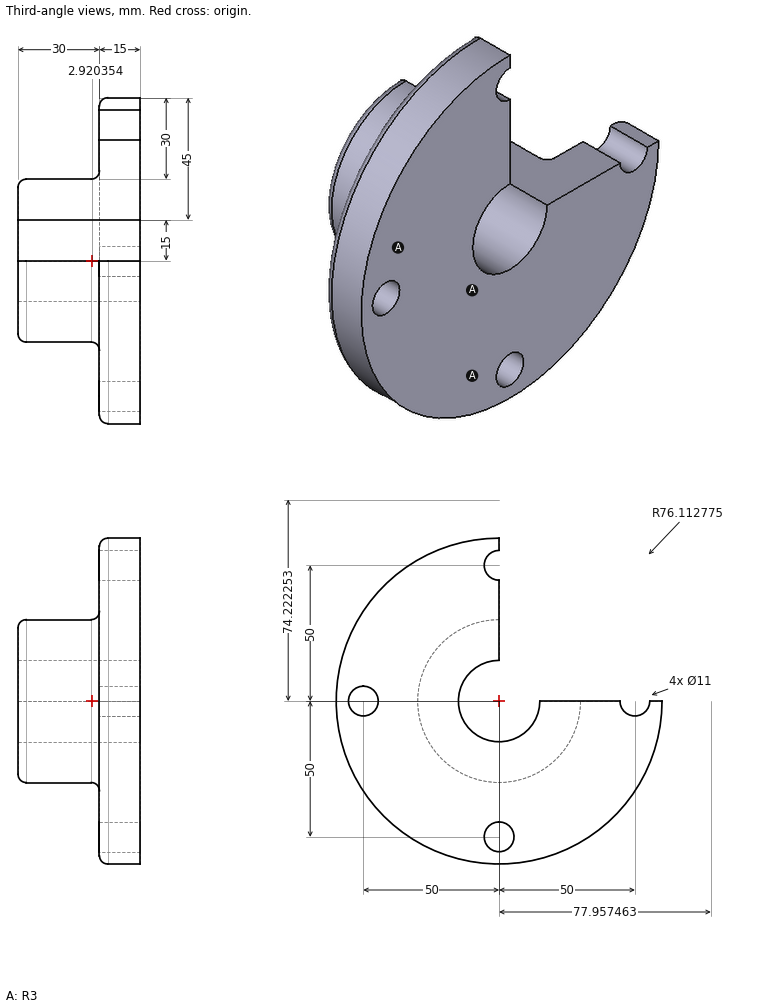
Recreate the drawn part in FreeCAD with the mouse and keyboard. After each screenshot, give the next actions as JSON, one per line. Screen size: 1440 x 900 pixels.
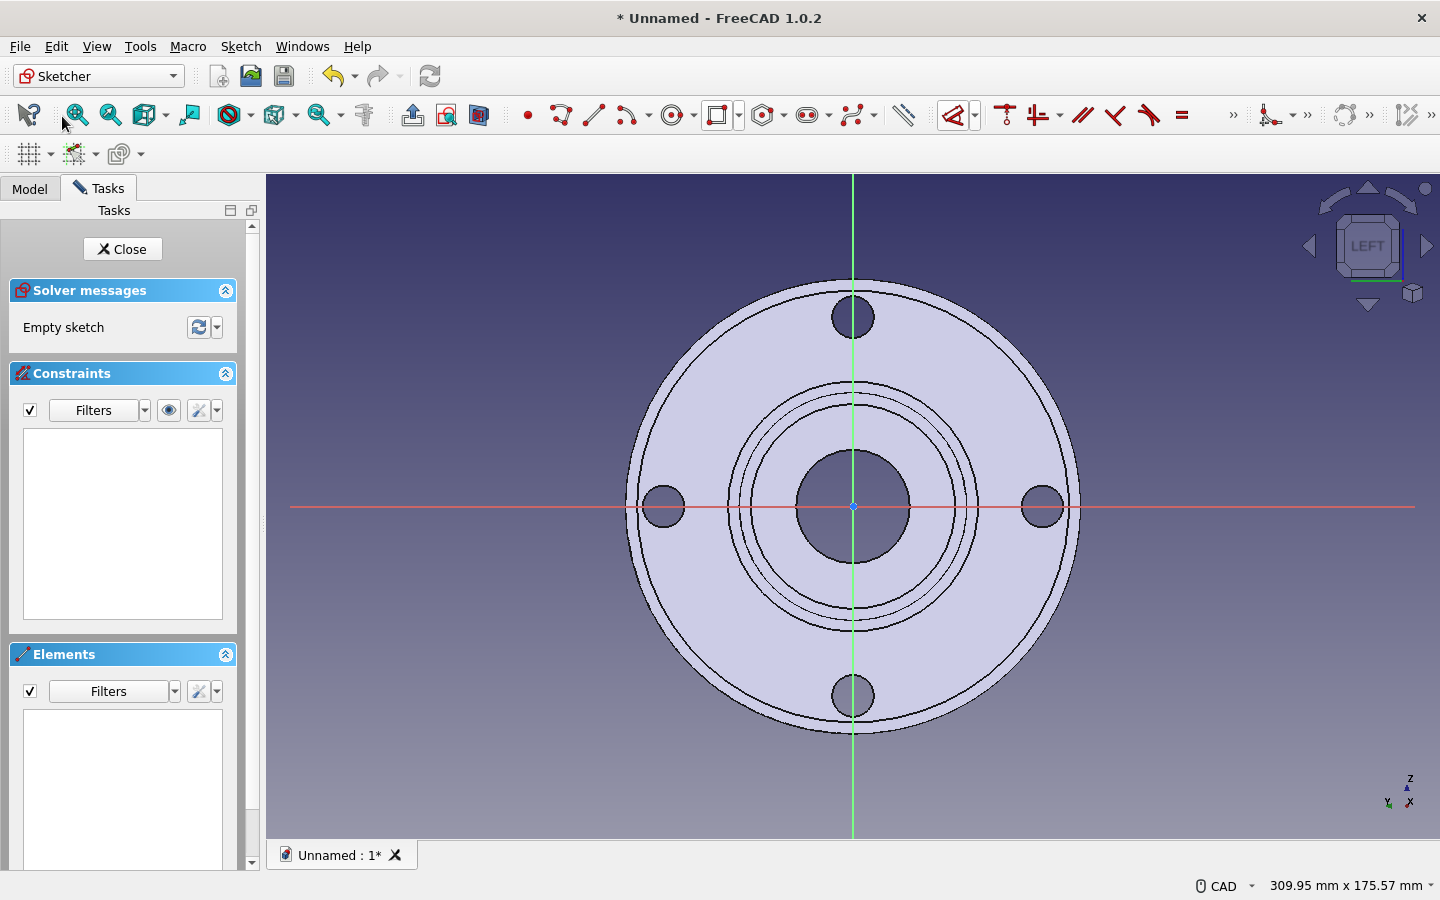
{"action": "scroll", "coordinate": [544, 202], "scroll_direction": "up", "scroll_amount": 2}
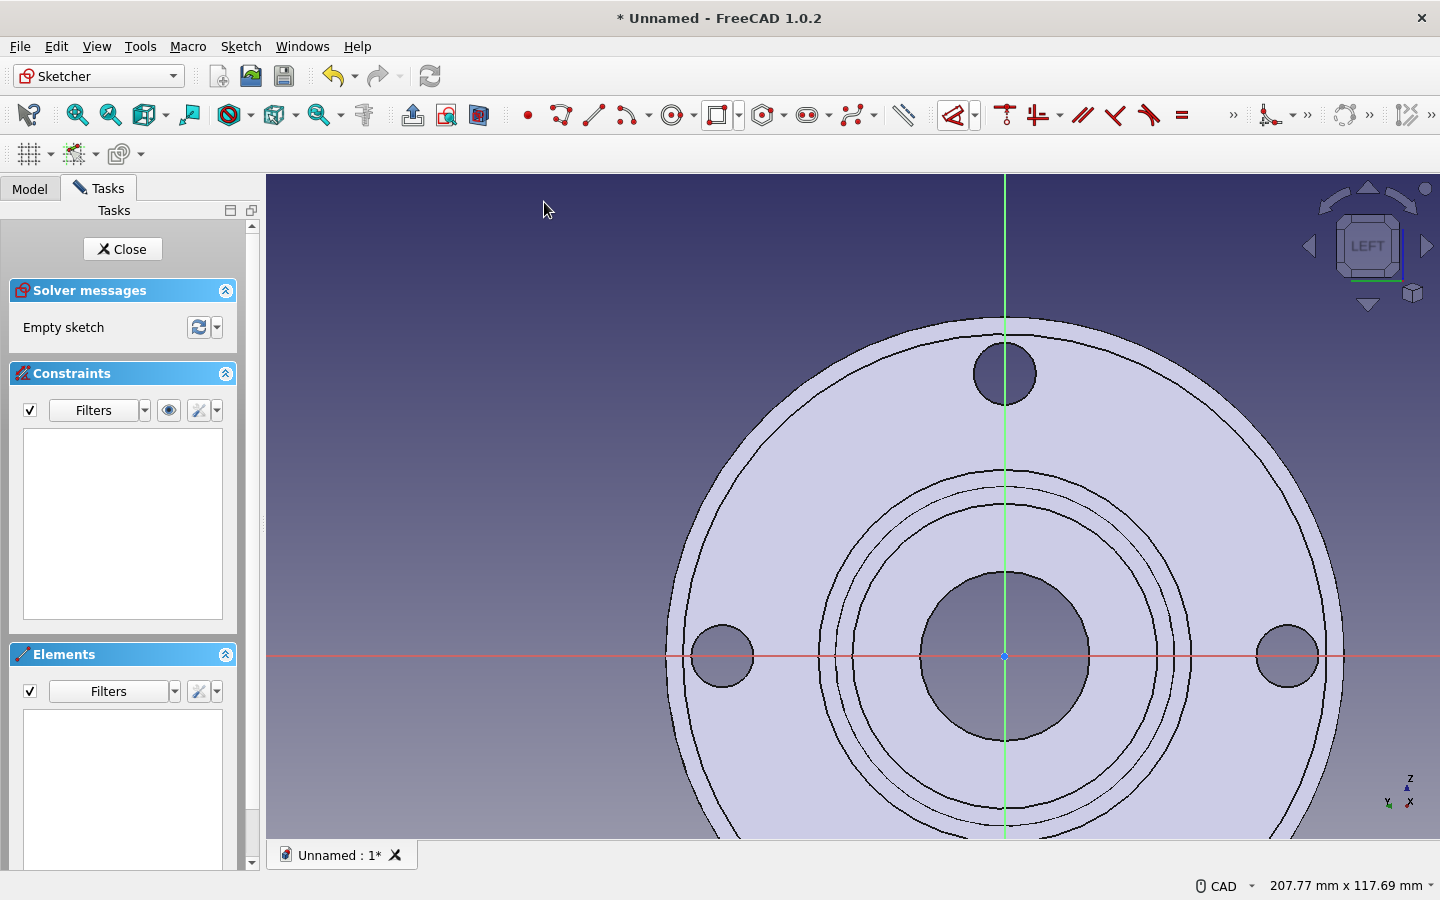
{"action": "left_click", "coordinate": [561, 116]}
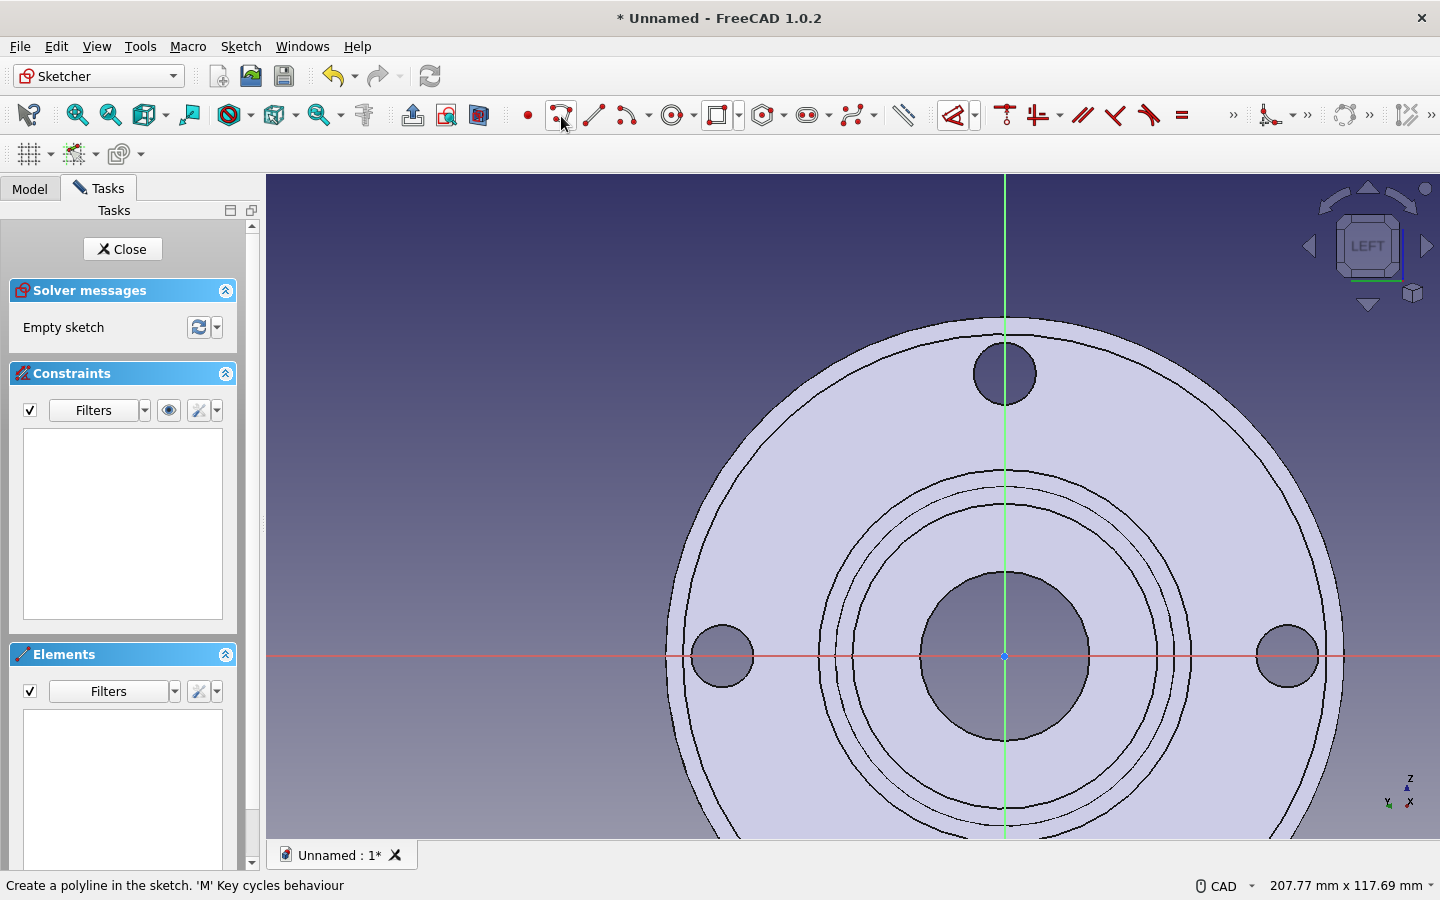
{"action": "left_click", "coordinate": [564, 656]}
{"action": "left_click", "coordinate": [1005, 656]}
{"action": "left_click", "coordinate": [996, 237]}
{"action": "right_click", "coordinate": [996, 237]}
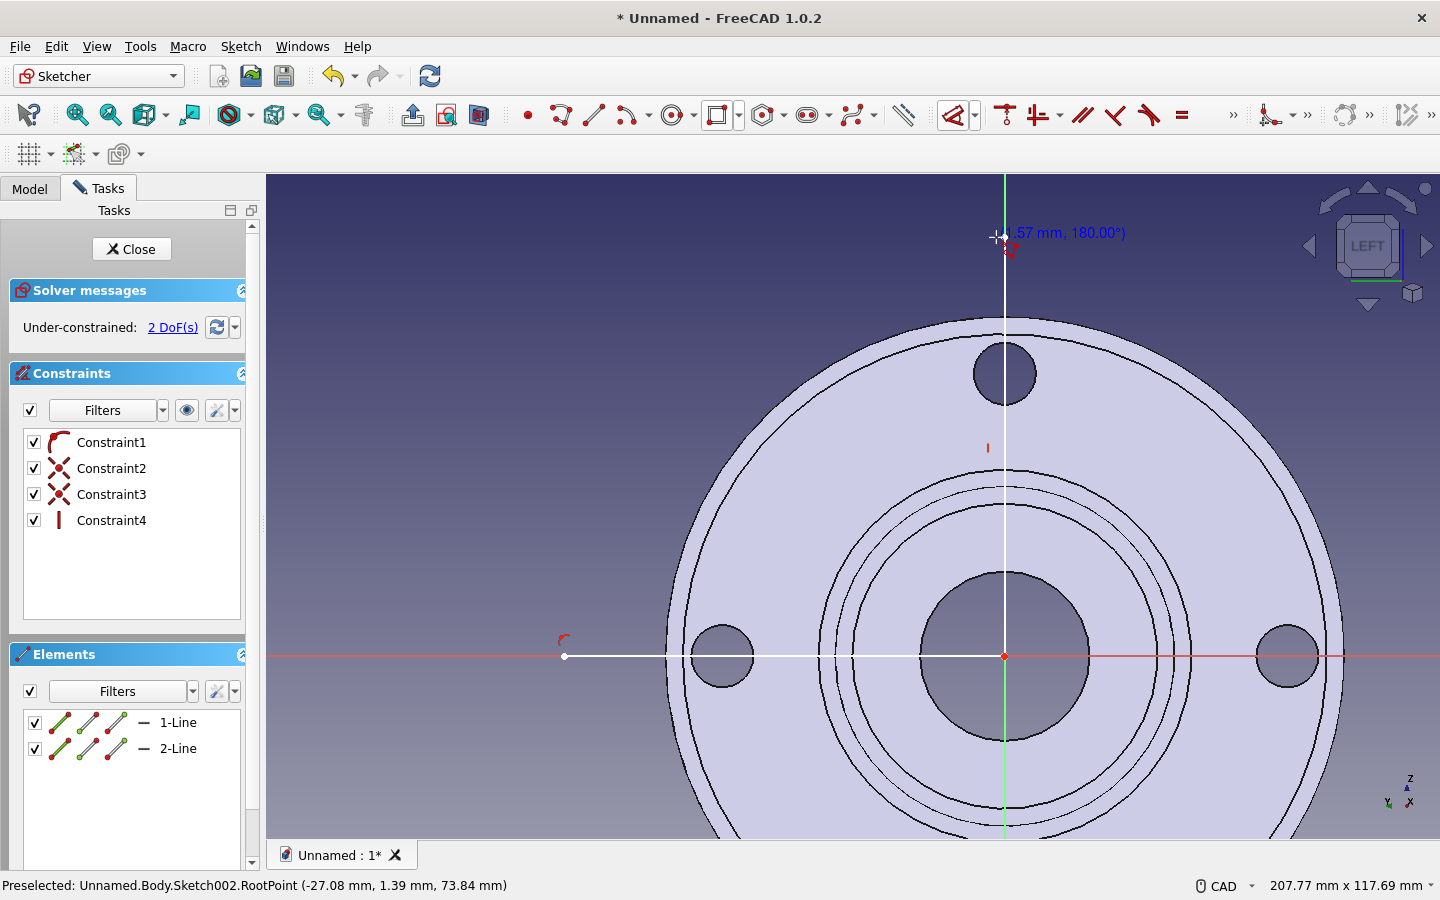
{"action": "left_click", "coordinate": [648, 116]}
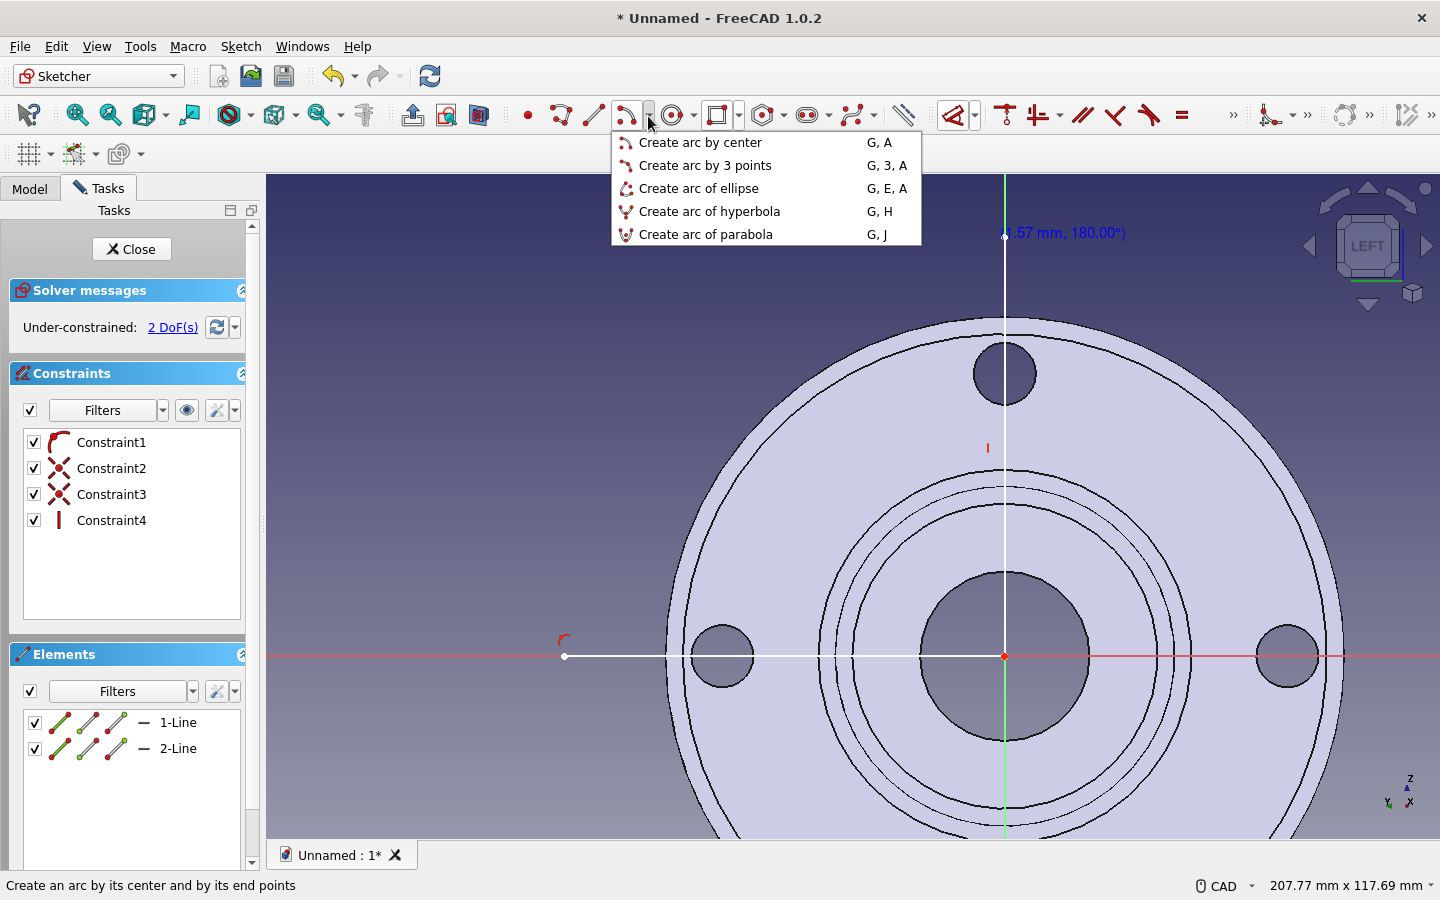
{"action": "left_click", "coordinate": [766, 166]}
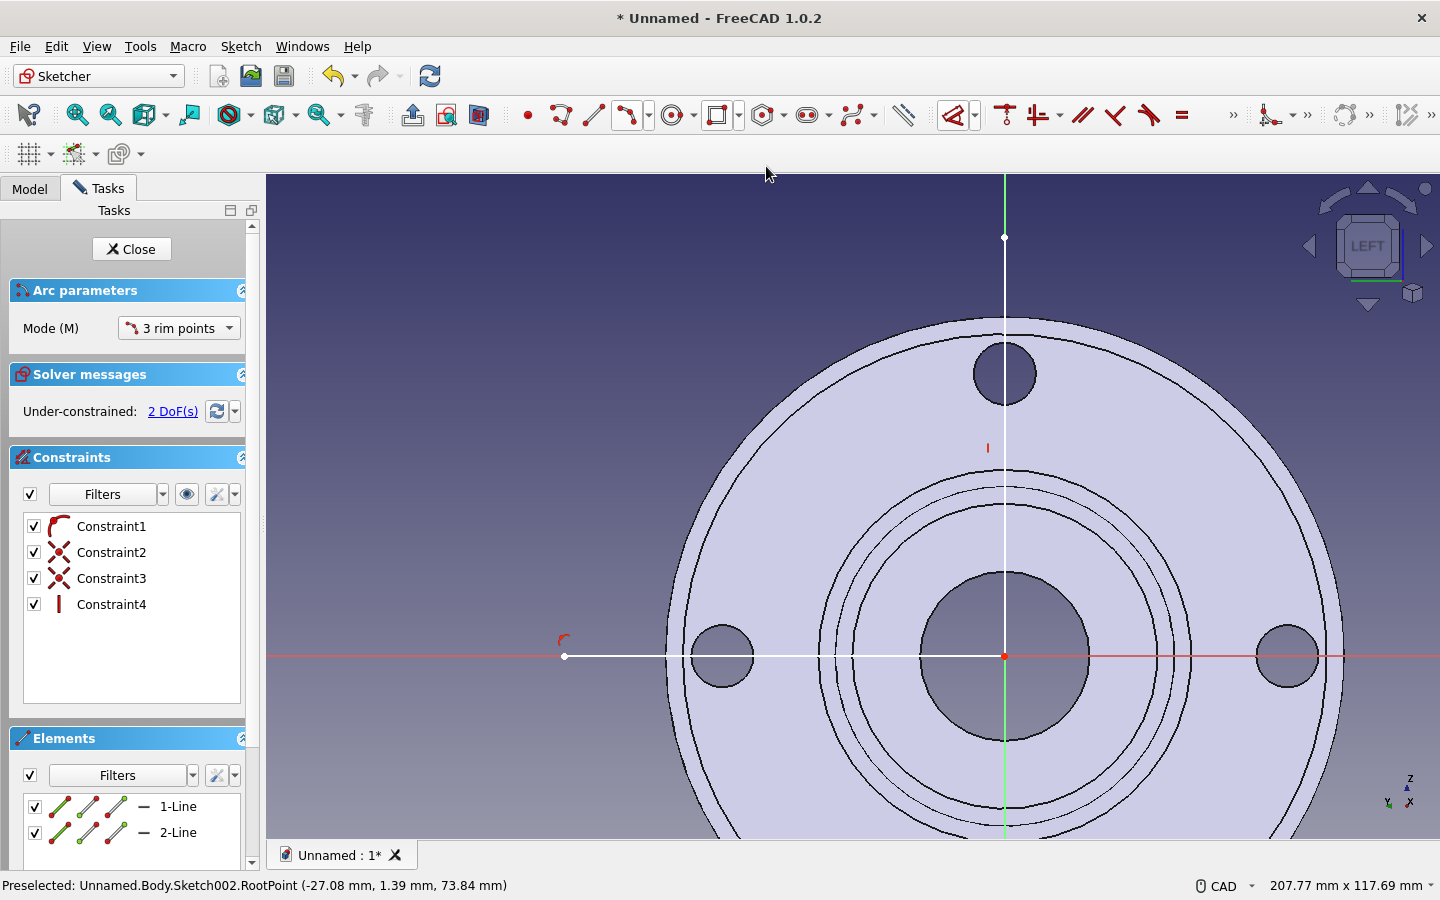
{"action": "left_click", "coordinate": [1005, 238]}
{"action": "left_click", "coordinate": [564, 656]}
{"action": "left_click", "coordinate": [698, 355]}
{"action": "key", "text": "Escape"}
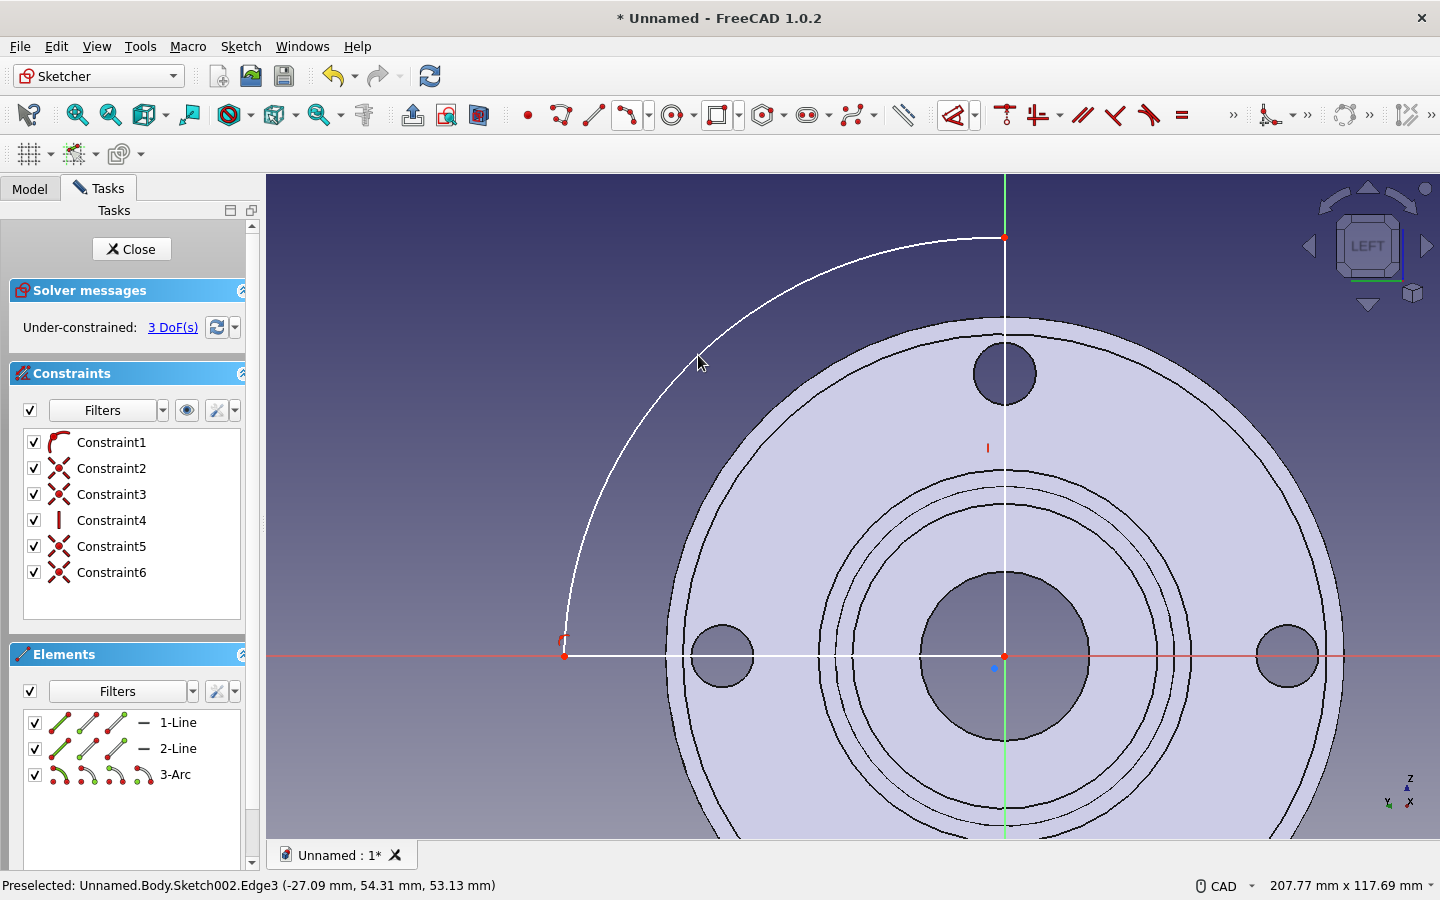
{"action": "left_click", "coordinate": [809, 280]}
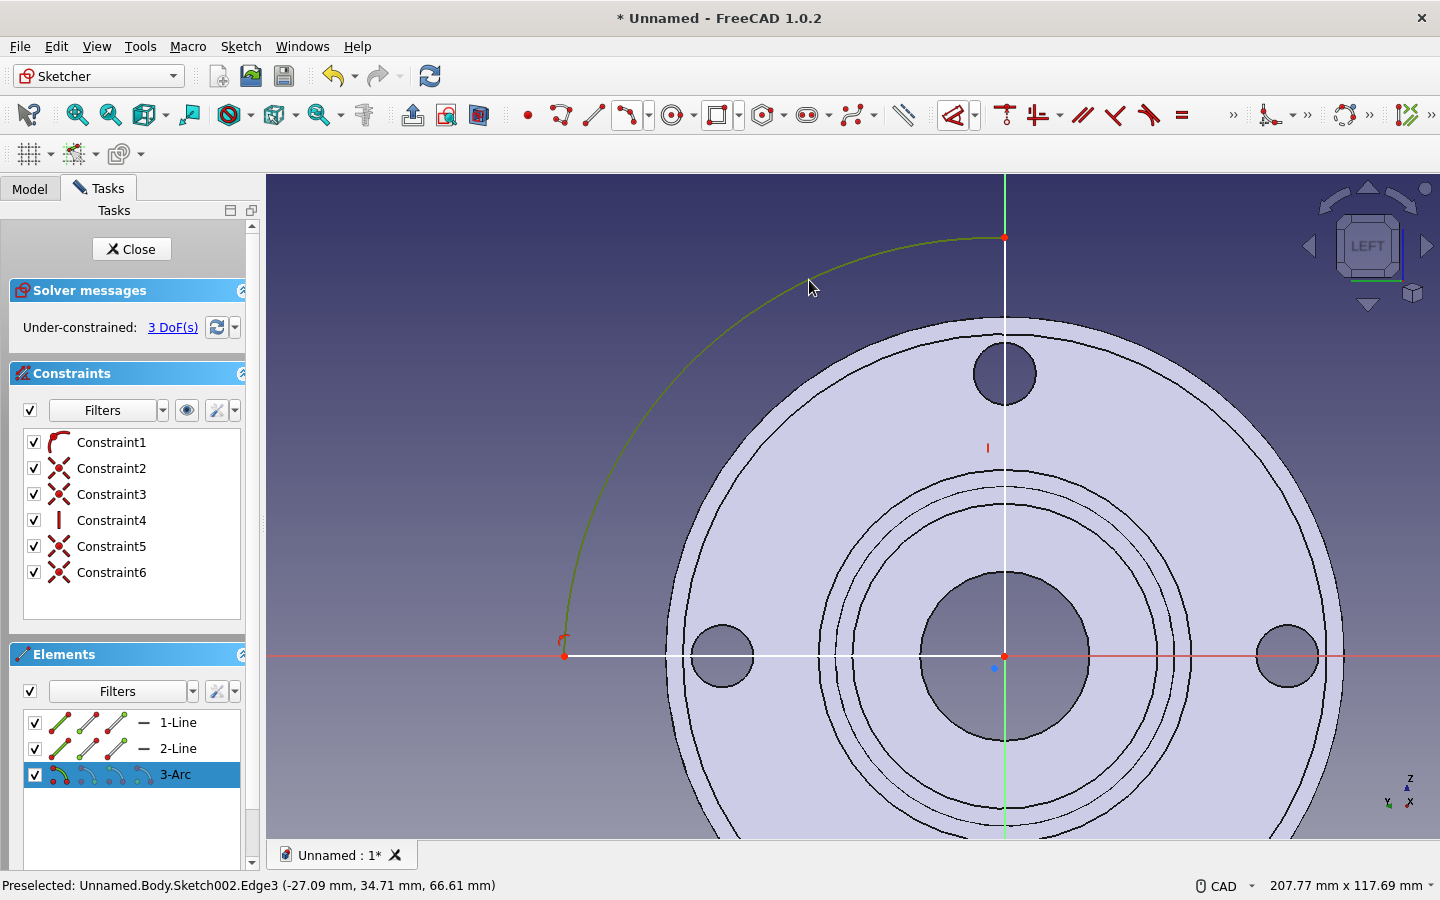
{"action": "key", "text": "k r"}